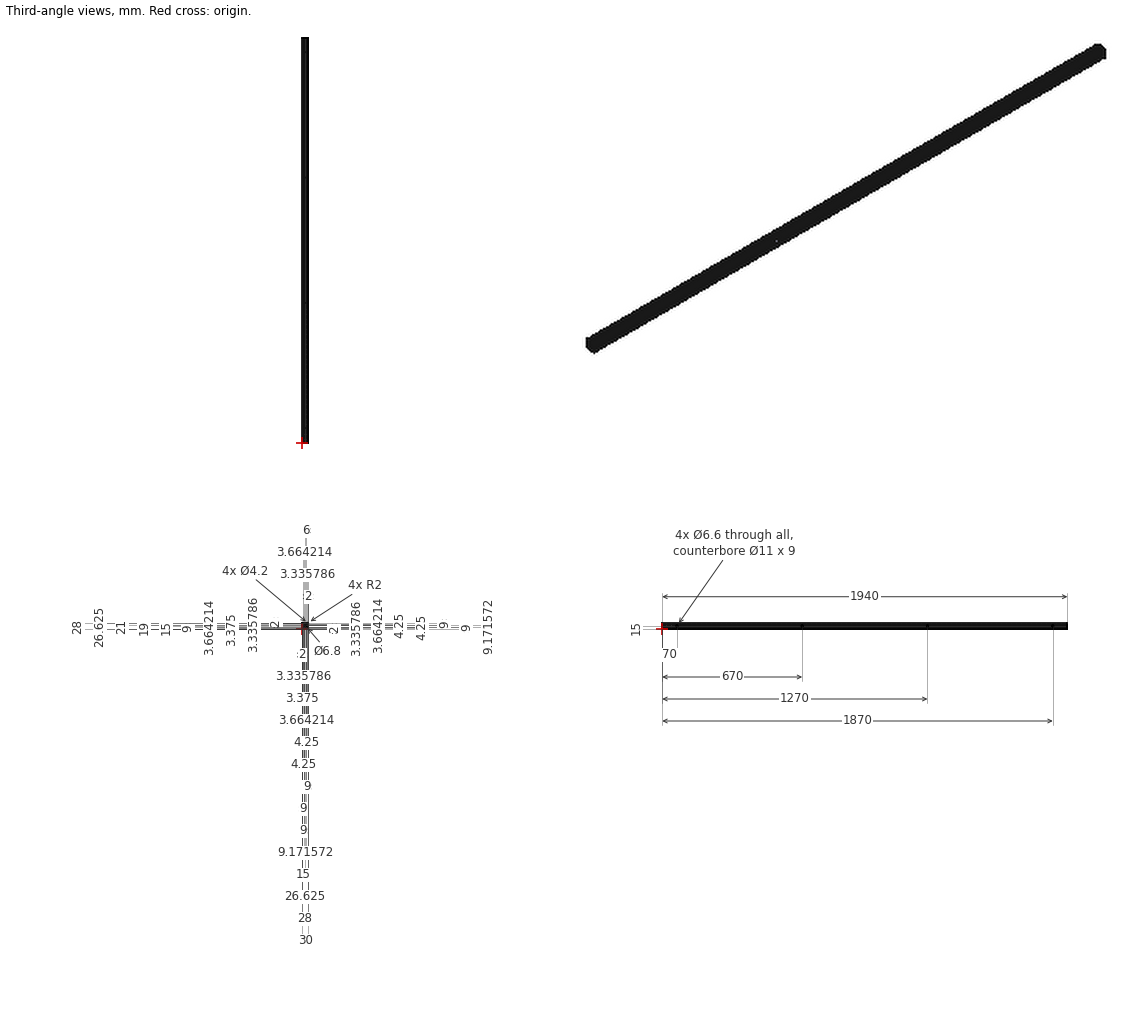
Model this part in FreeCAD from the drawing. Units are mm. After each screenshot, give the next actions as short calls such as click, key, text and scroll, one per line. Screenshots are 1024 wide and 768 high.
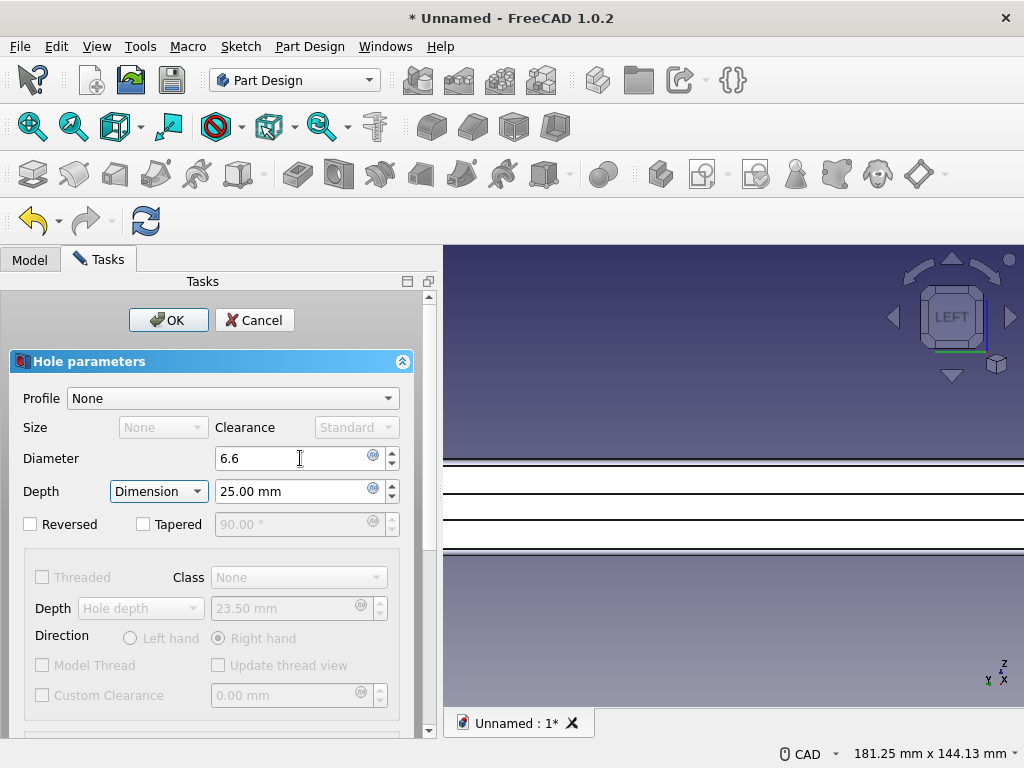
click(160, 492)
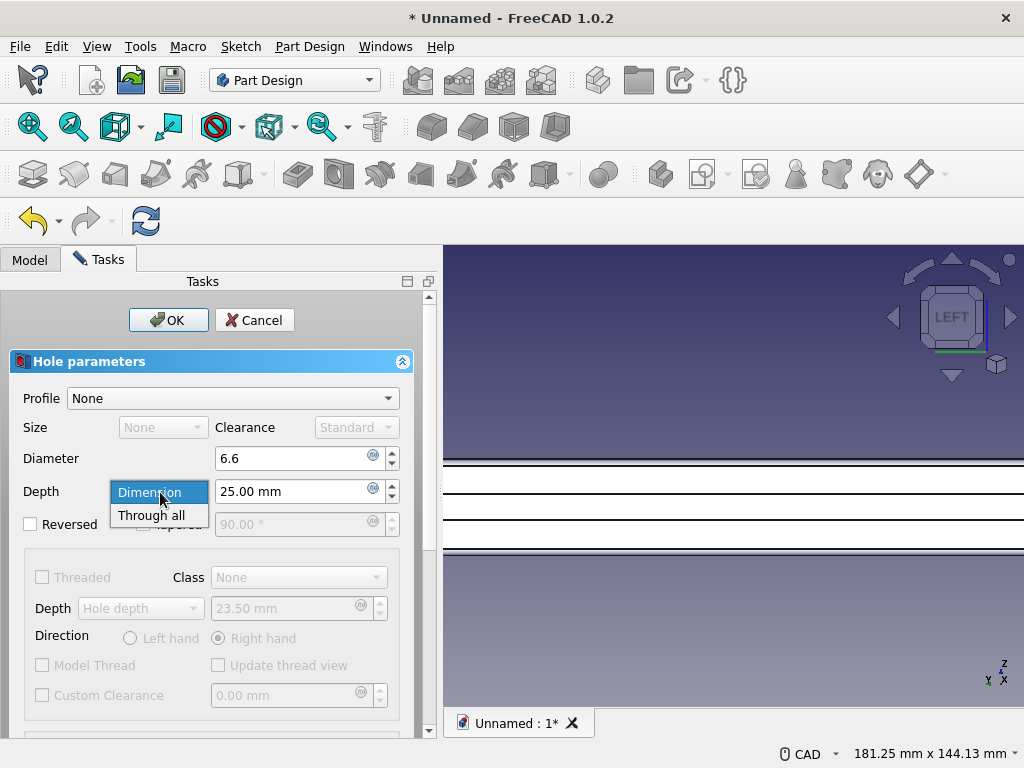
click(158, 516)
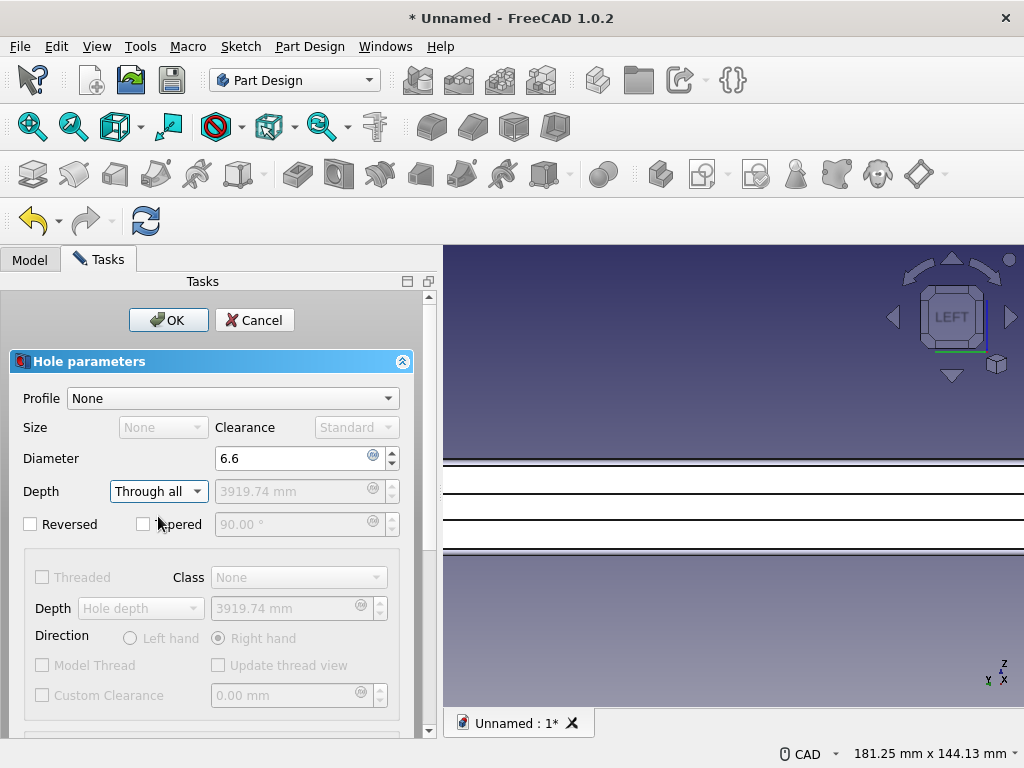
scroll(429, 514, down, 2)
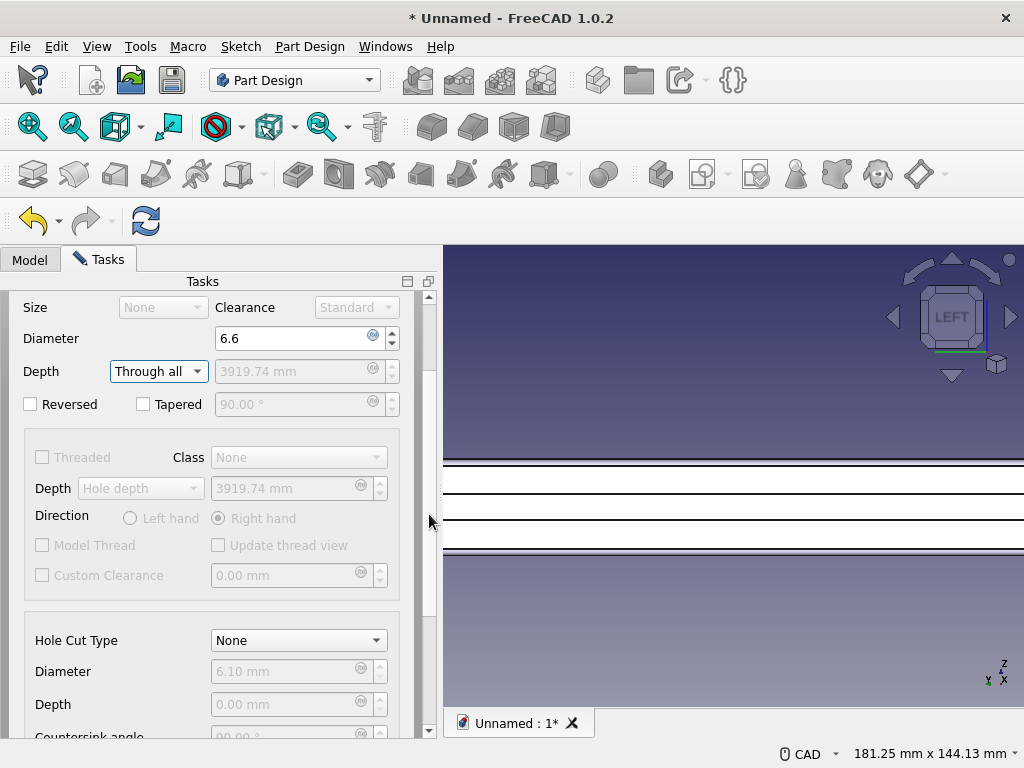
click(300, 640)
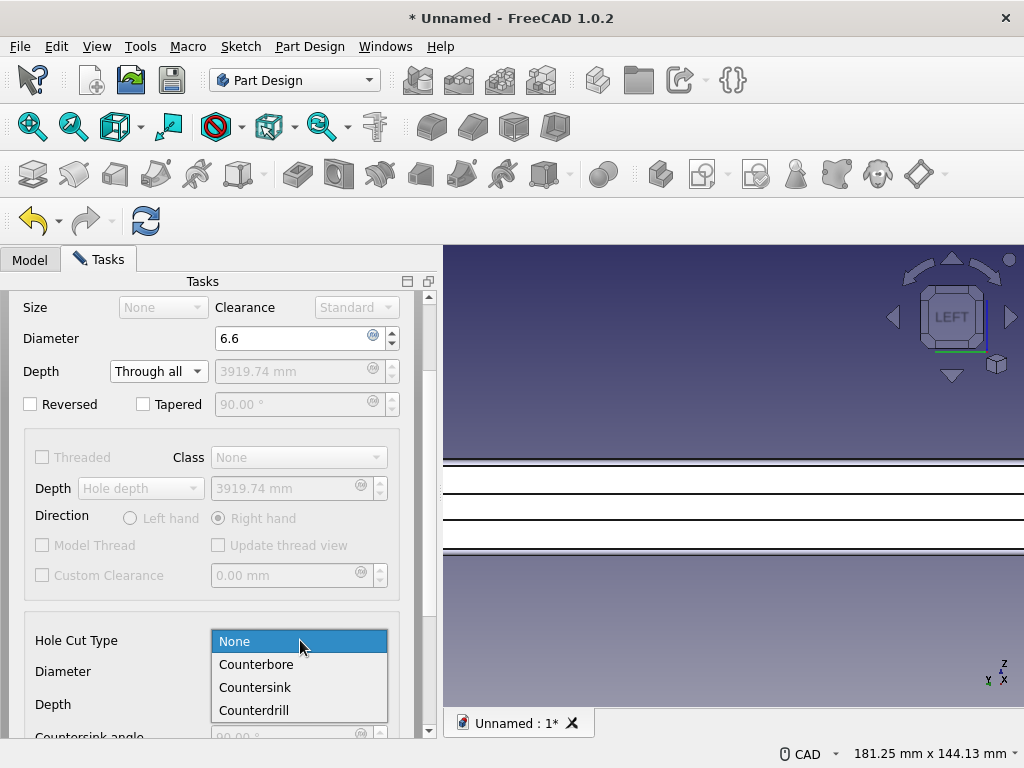
click(298, 664)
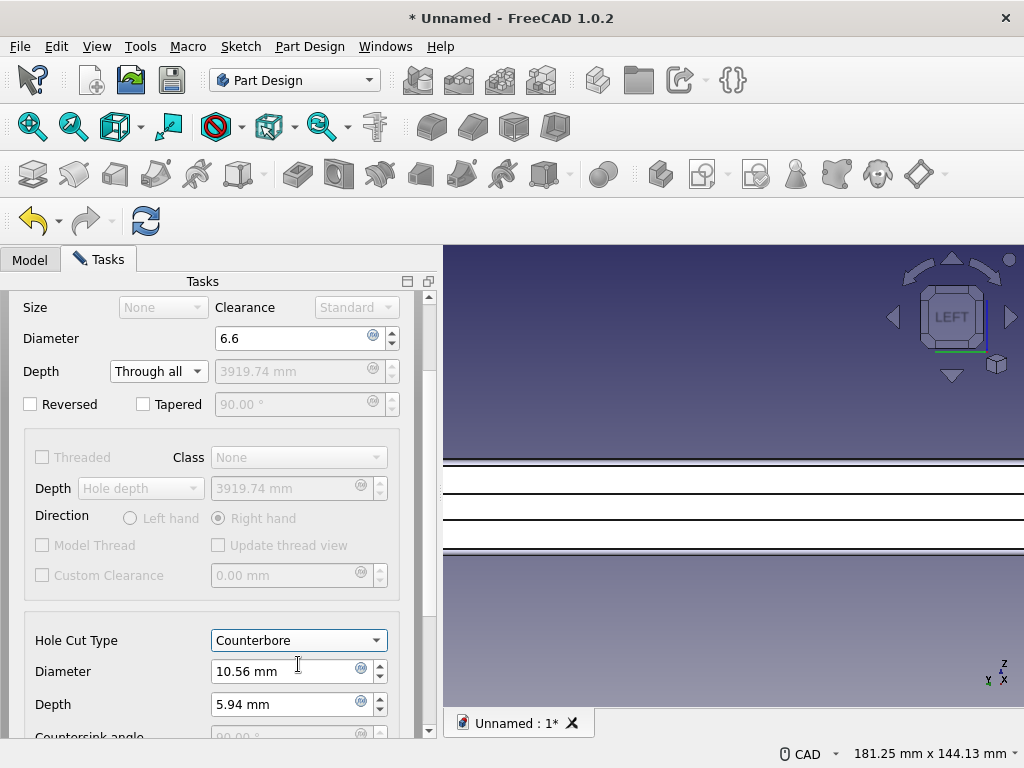
triple_click(292, 672)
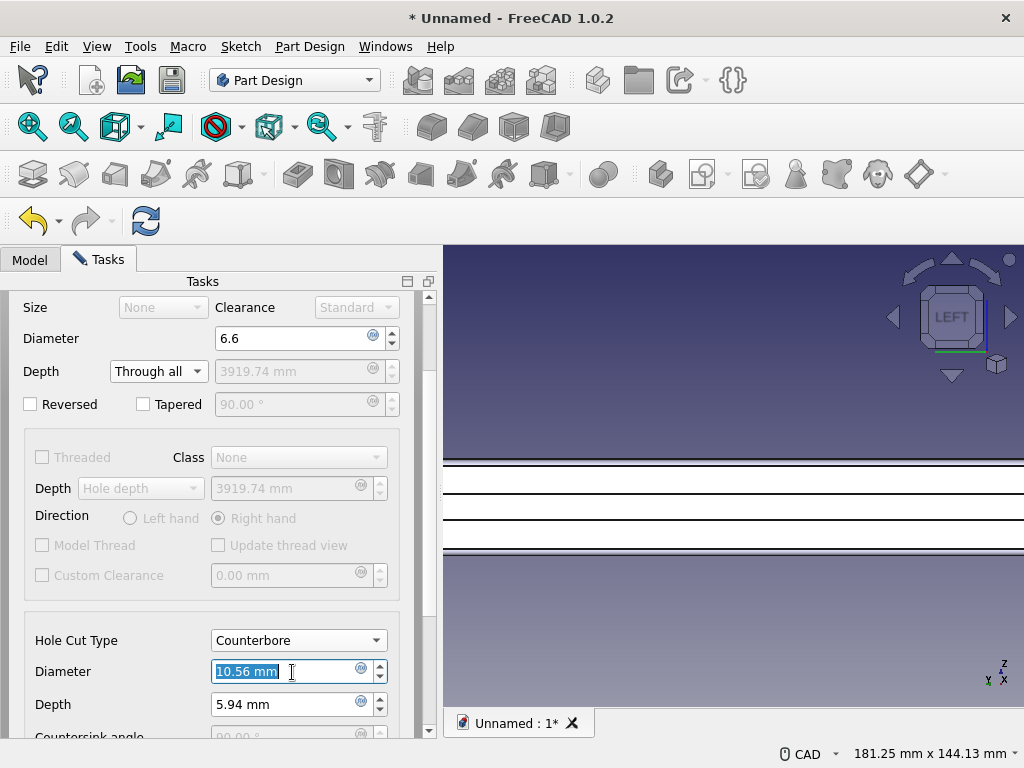
text(11)
key(Tab)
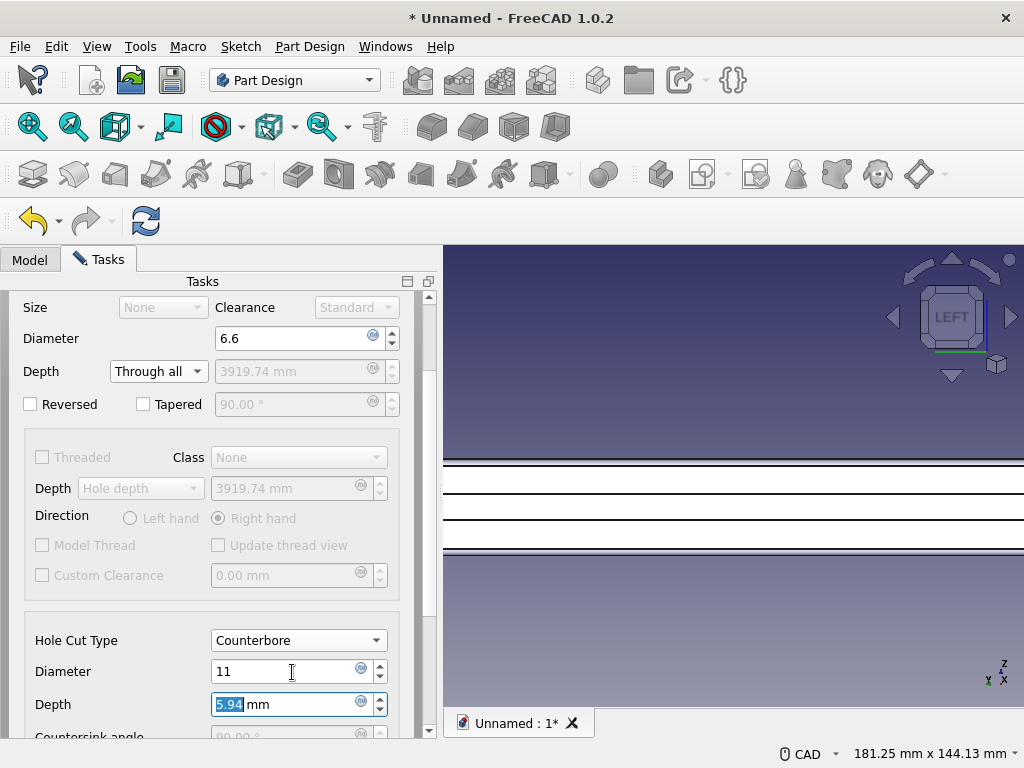
text(9)
key(Tab)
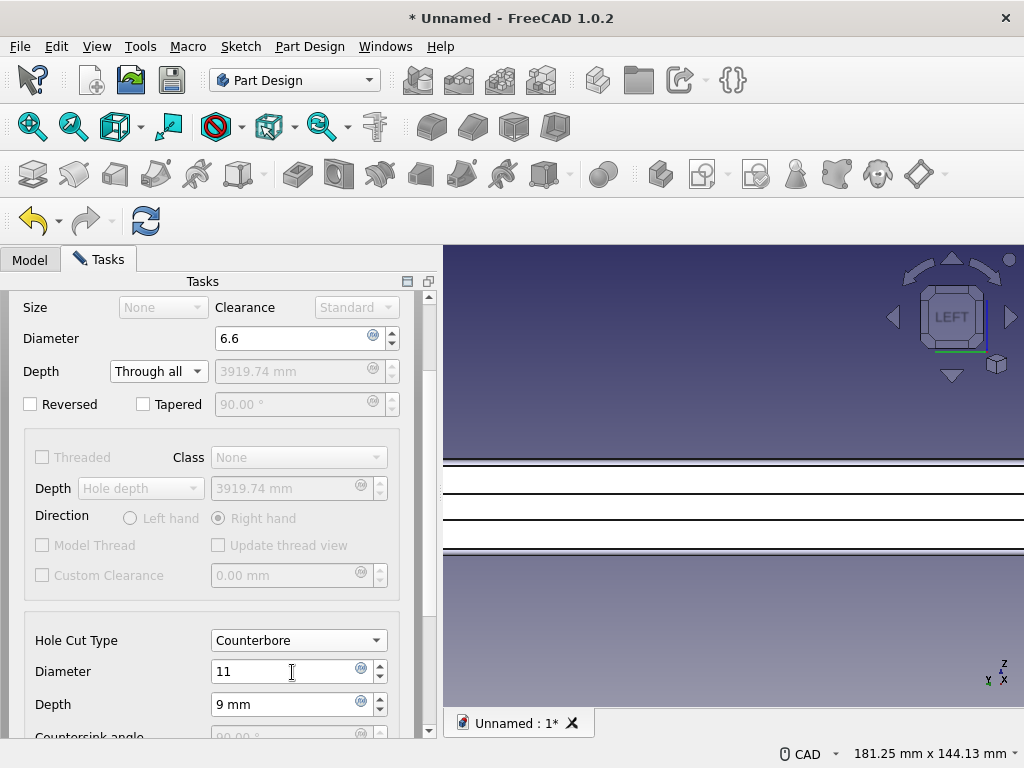
scroll(429, 514, up, 3)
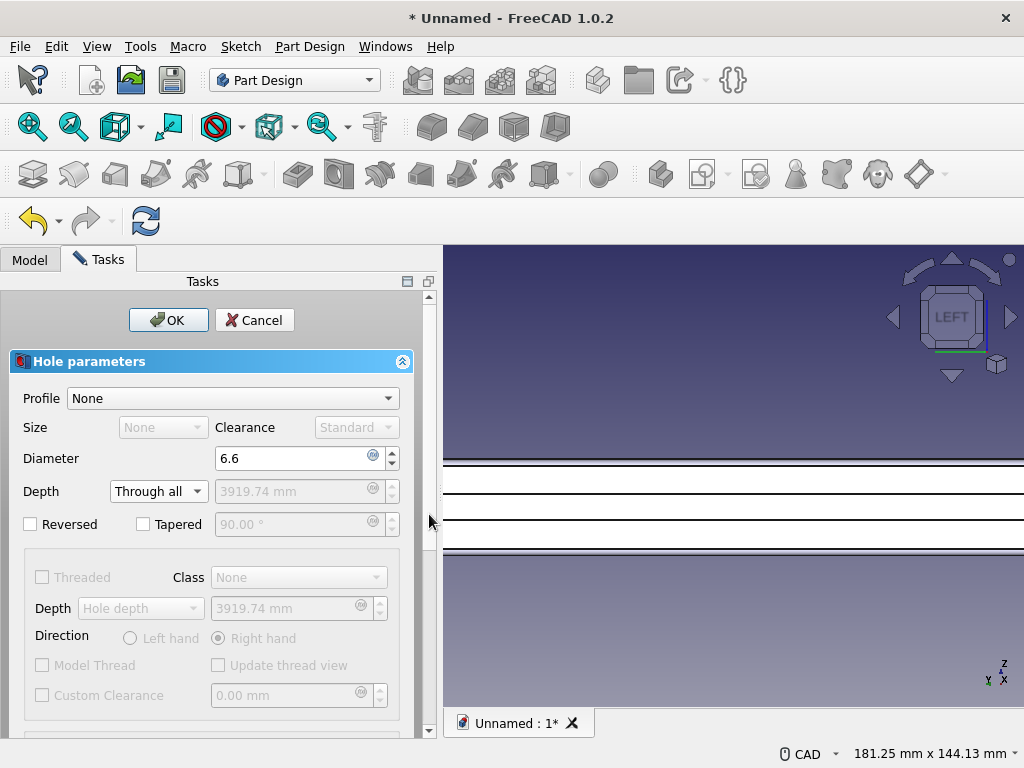
click(169, 320)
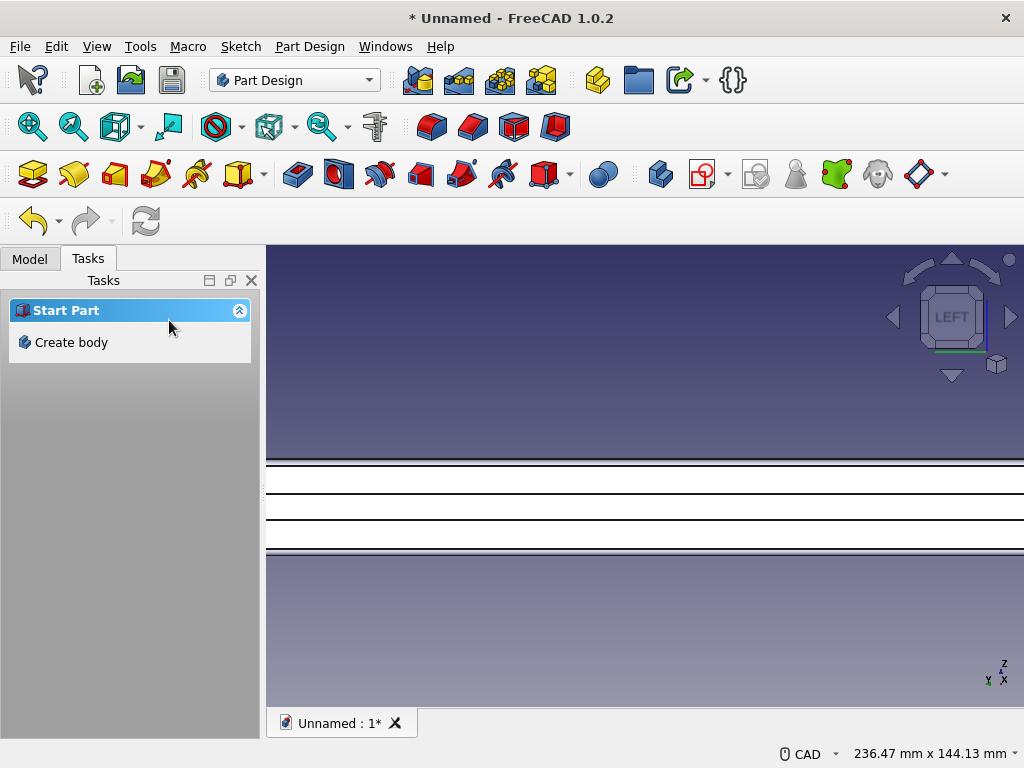
key(0)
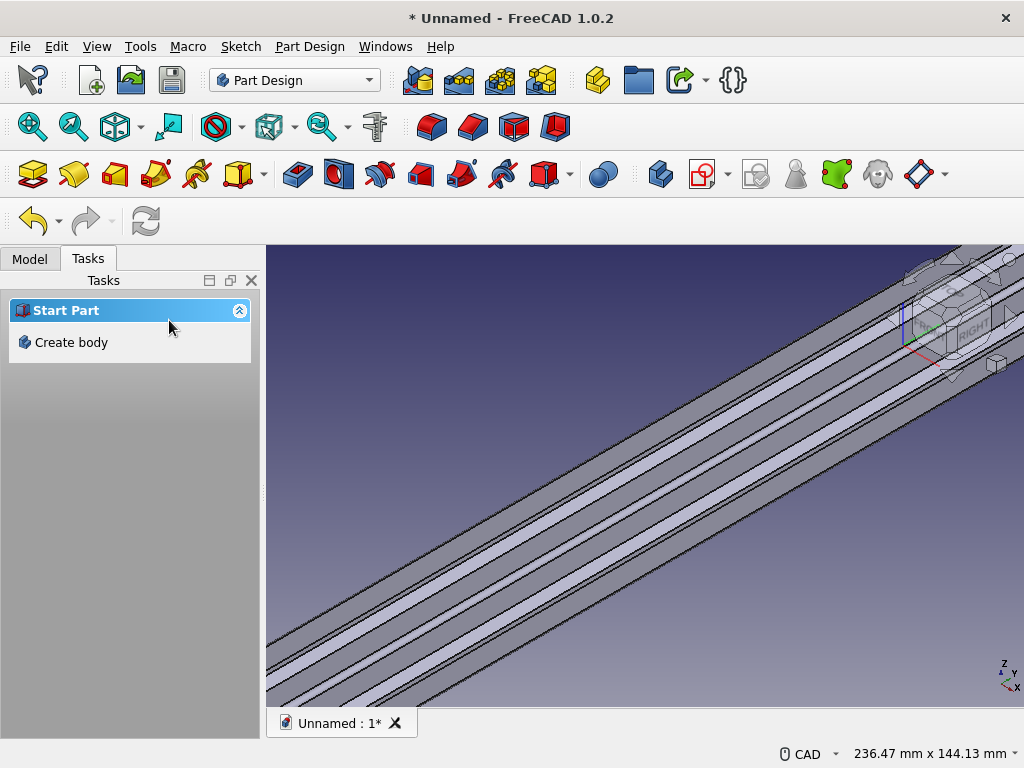
key(v)
key(f)